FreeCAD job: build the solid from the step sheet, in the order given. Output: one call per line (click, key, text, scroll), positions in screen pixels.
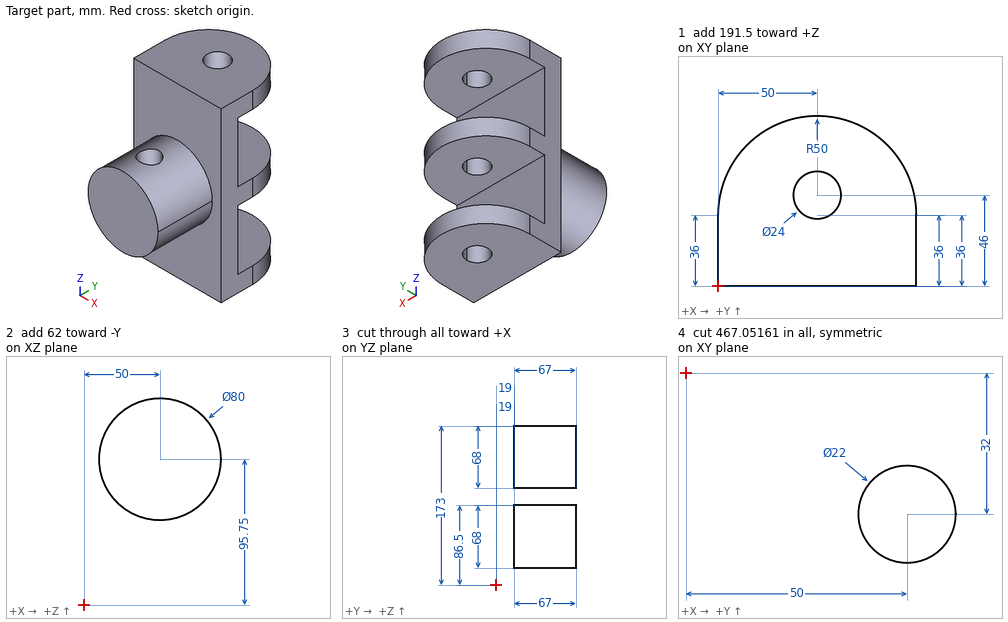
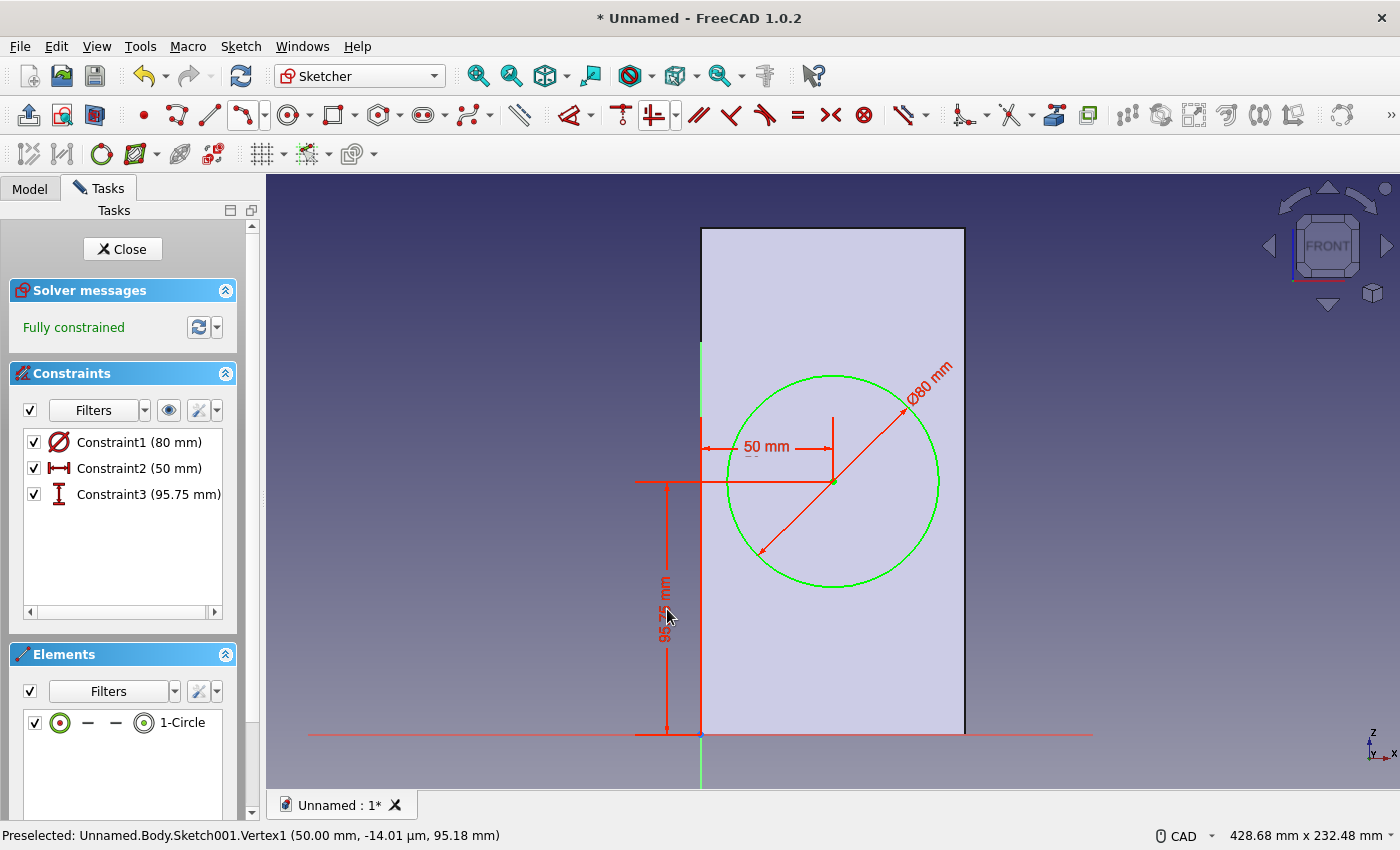
click(123, 249)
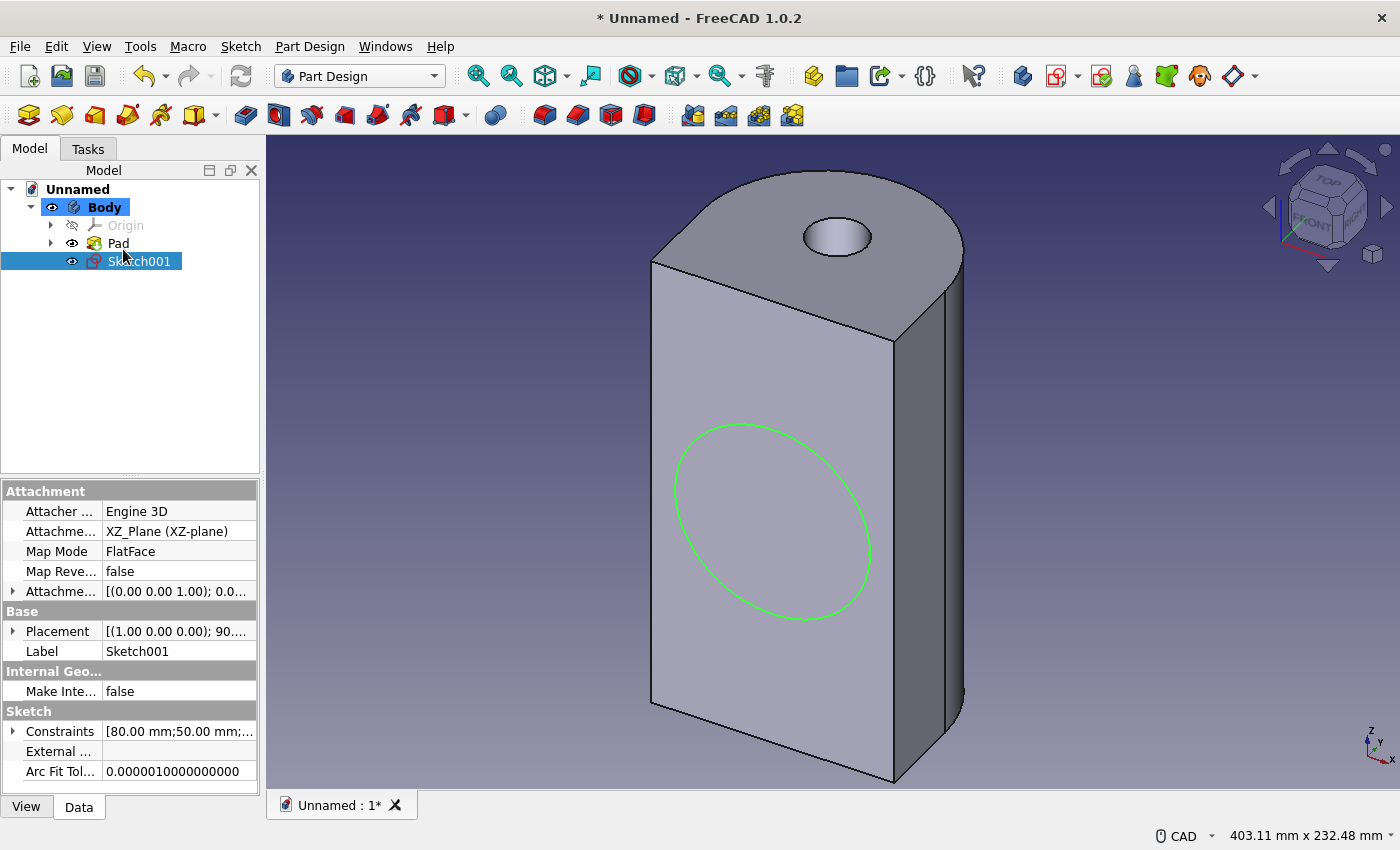
click(29, 116)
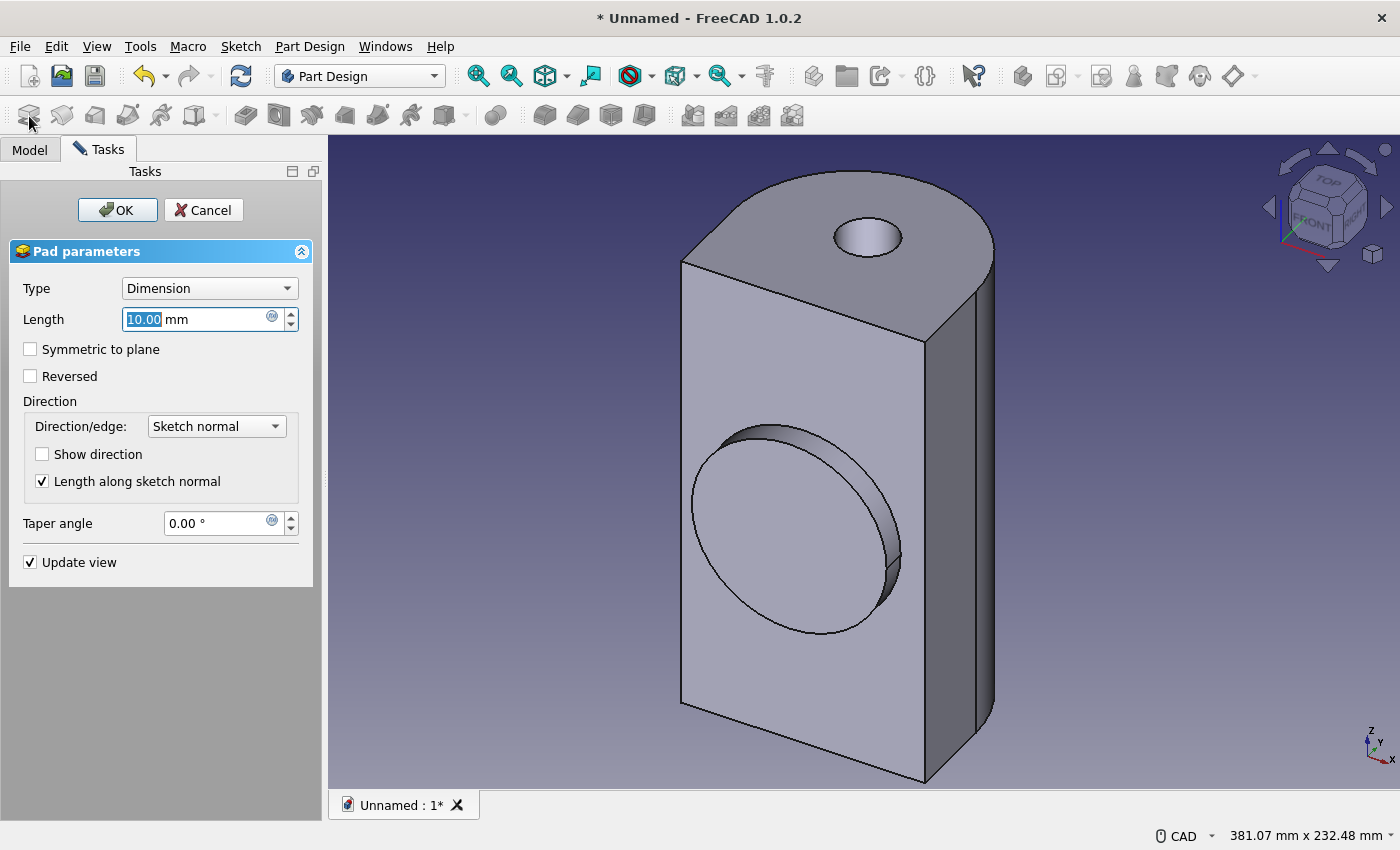
text(62)
key(Tab)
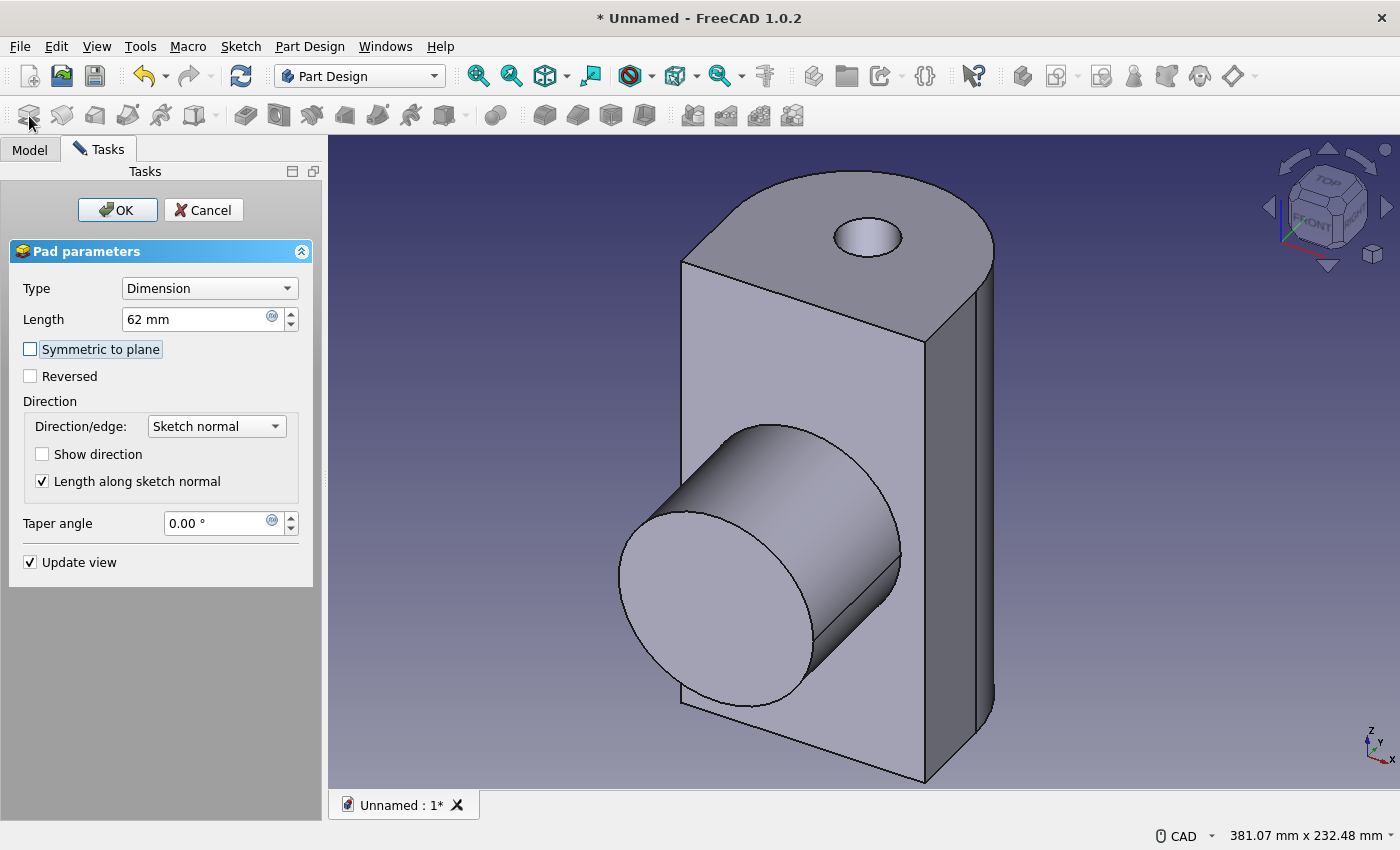
click(118, 210)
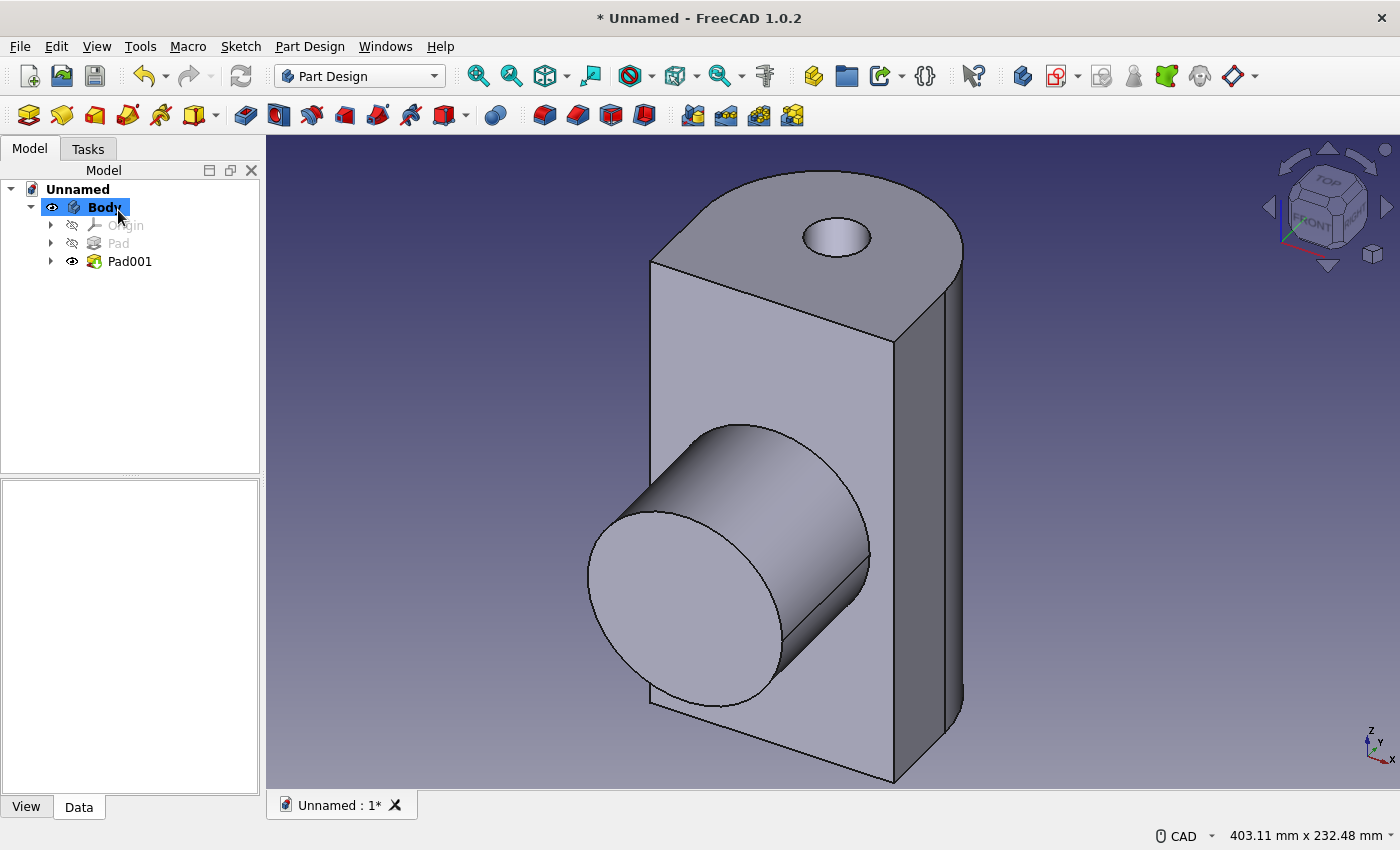
click(479, 76)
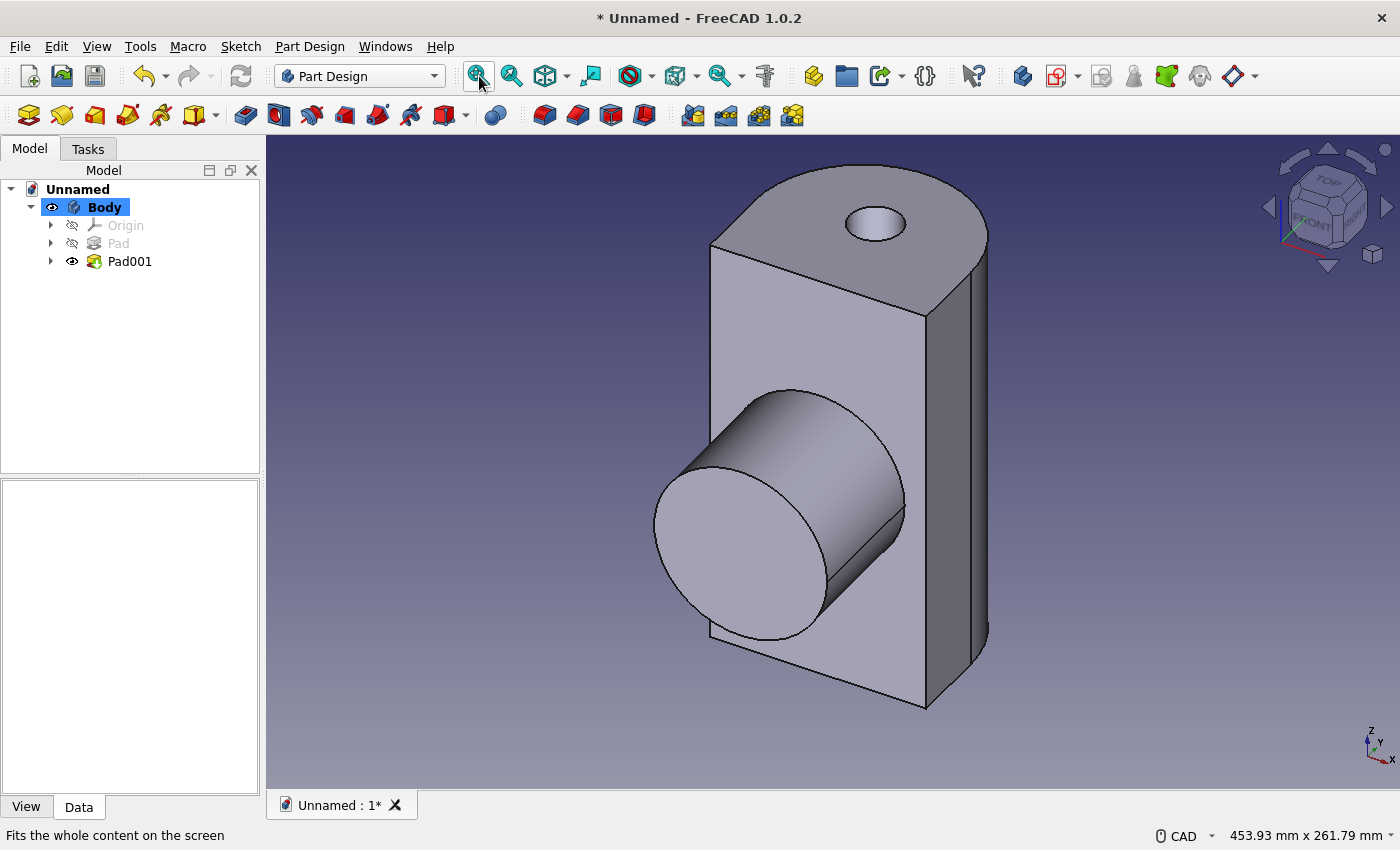
click(1056, 76)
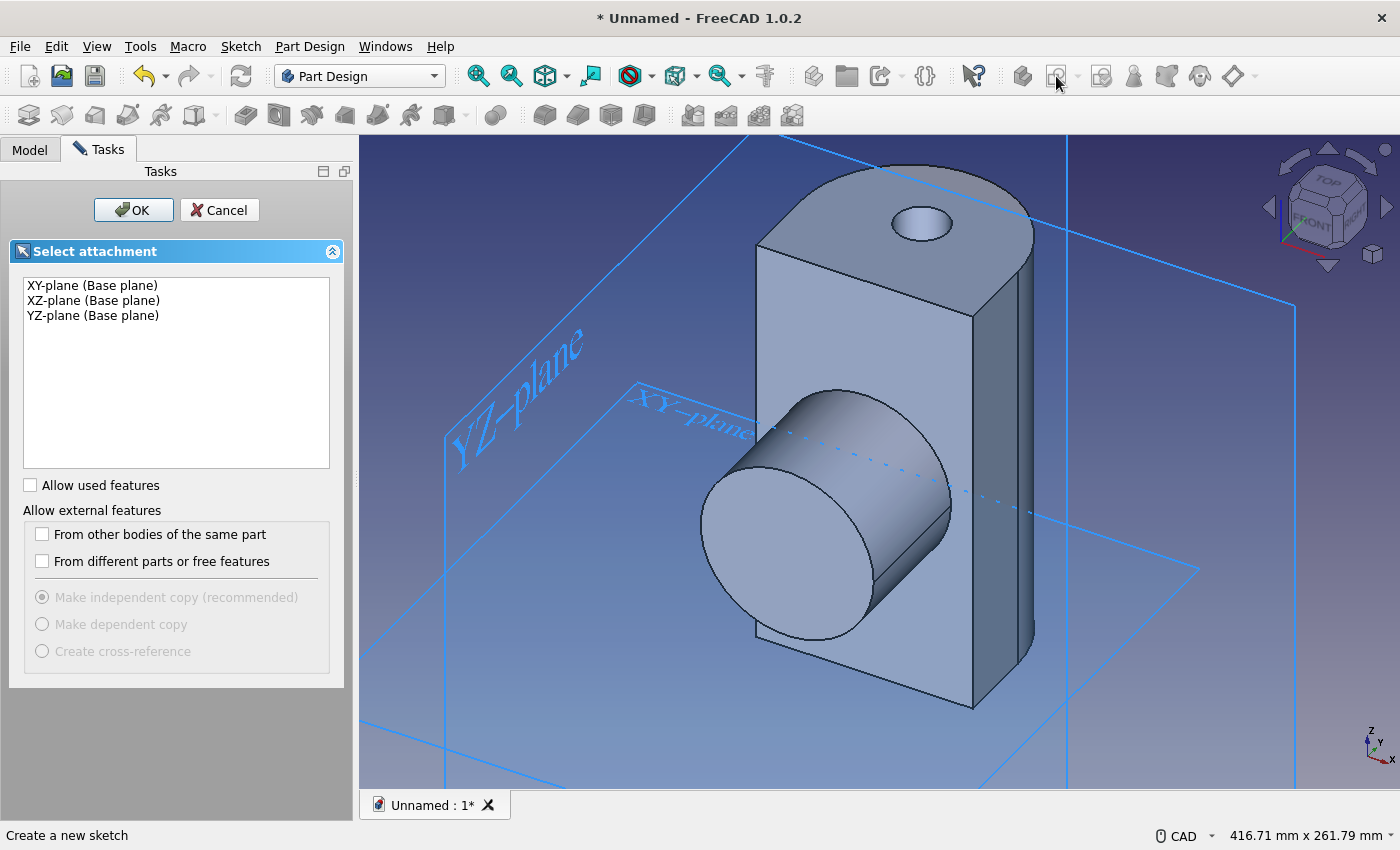
click(84, 316)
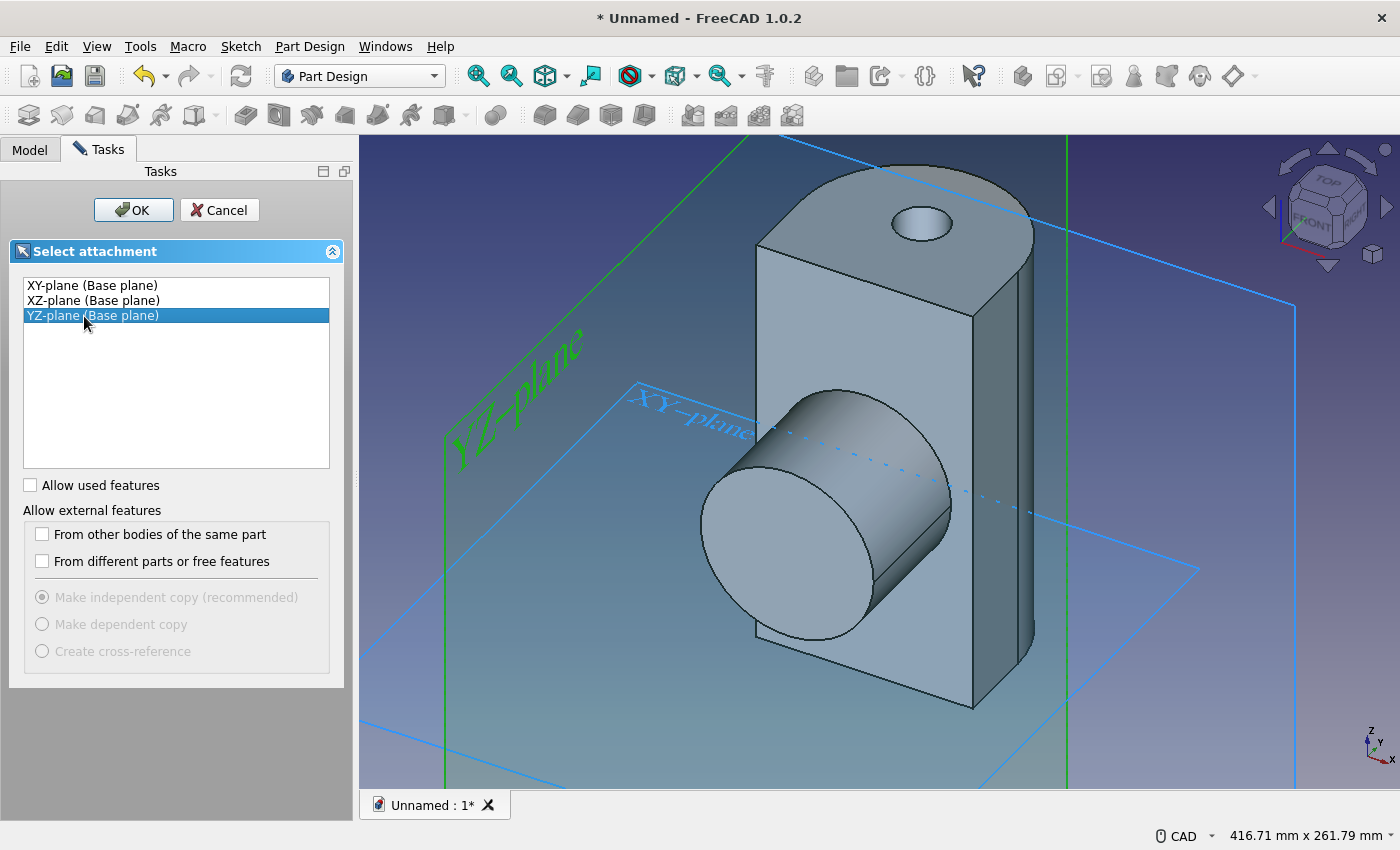
click(134, 210)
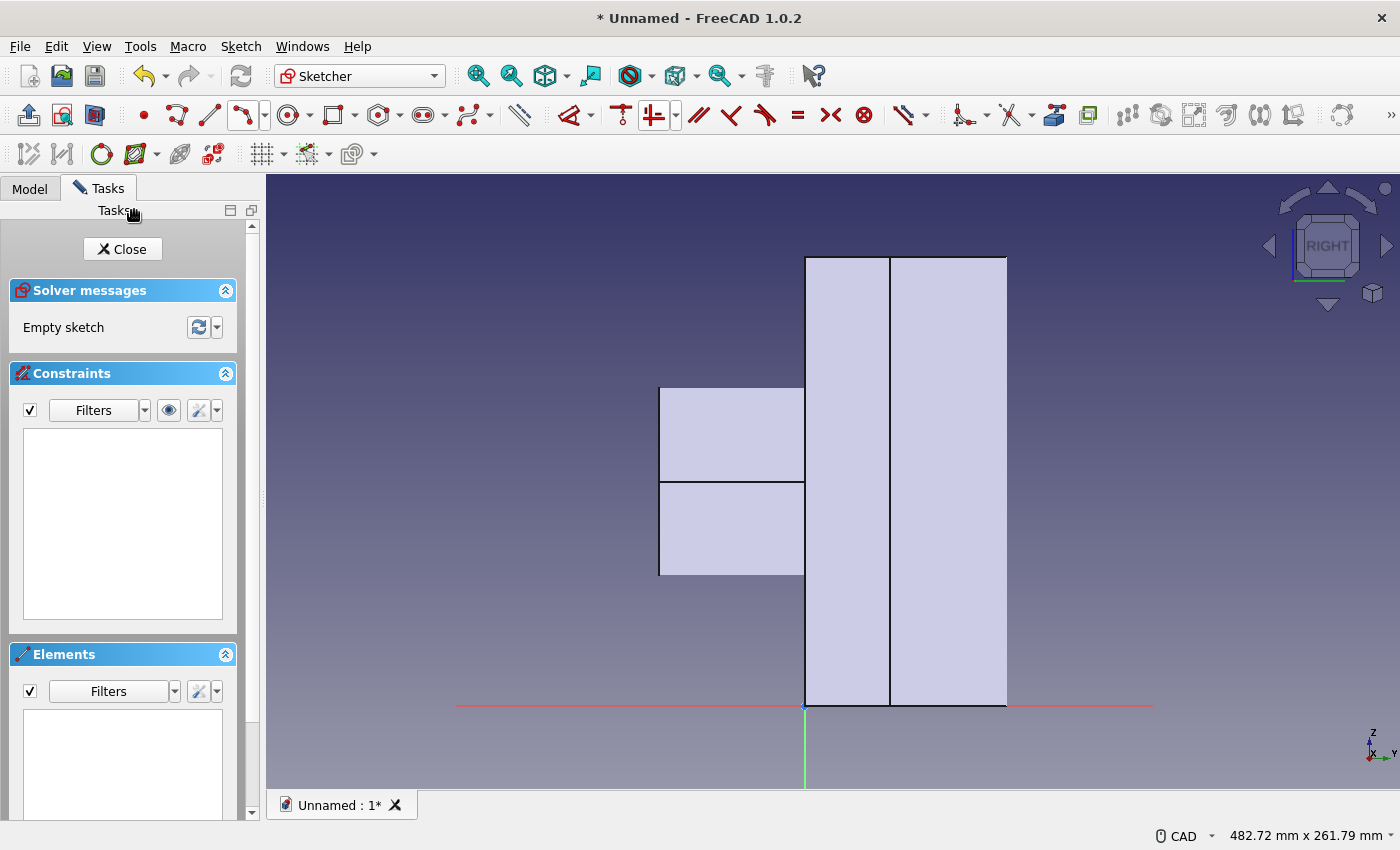
click(95, 116)